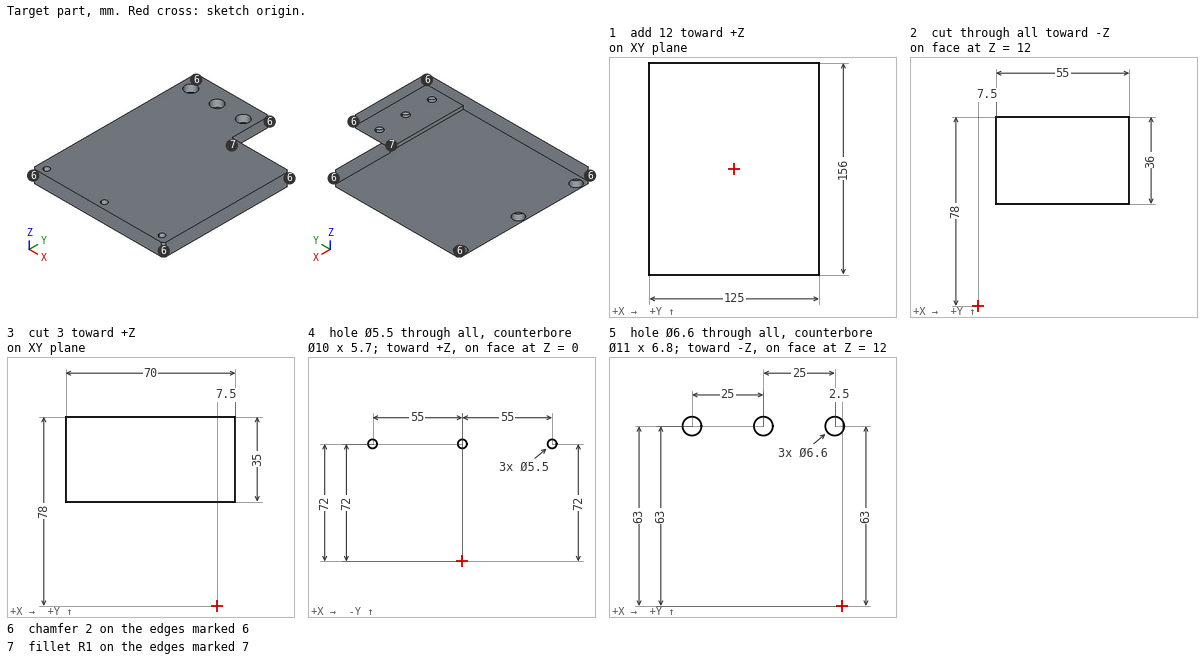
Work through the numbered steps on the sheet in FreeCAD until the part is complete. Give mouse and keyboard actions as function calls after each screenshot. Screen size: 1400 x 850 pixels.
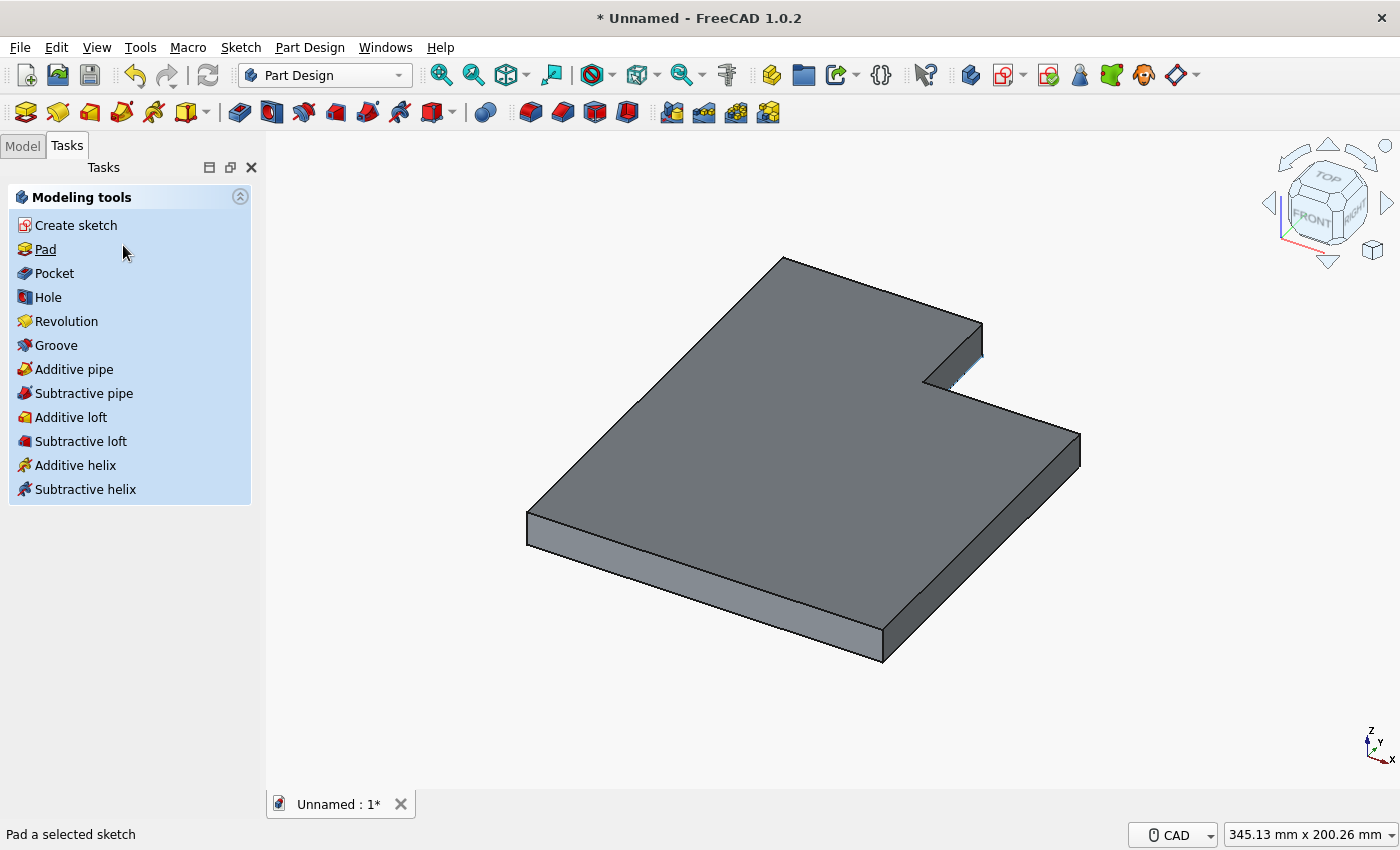
click(240, 112)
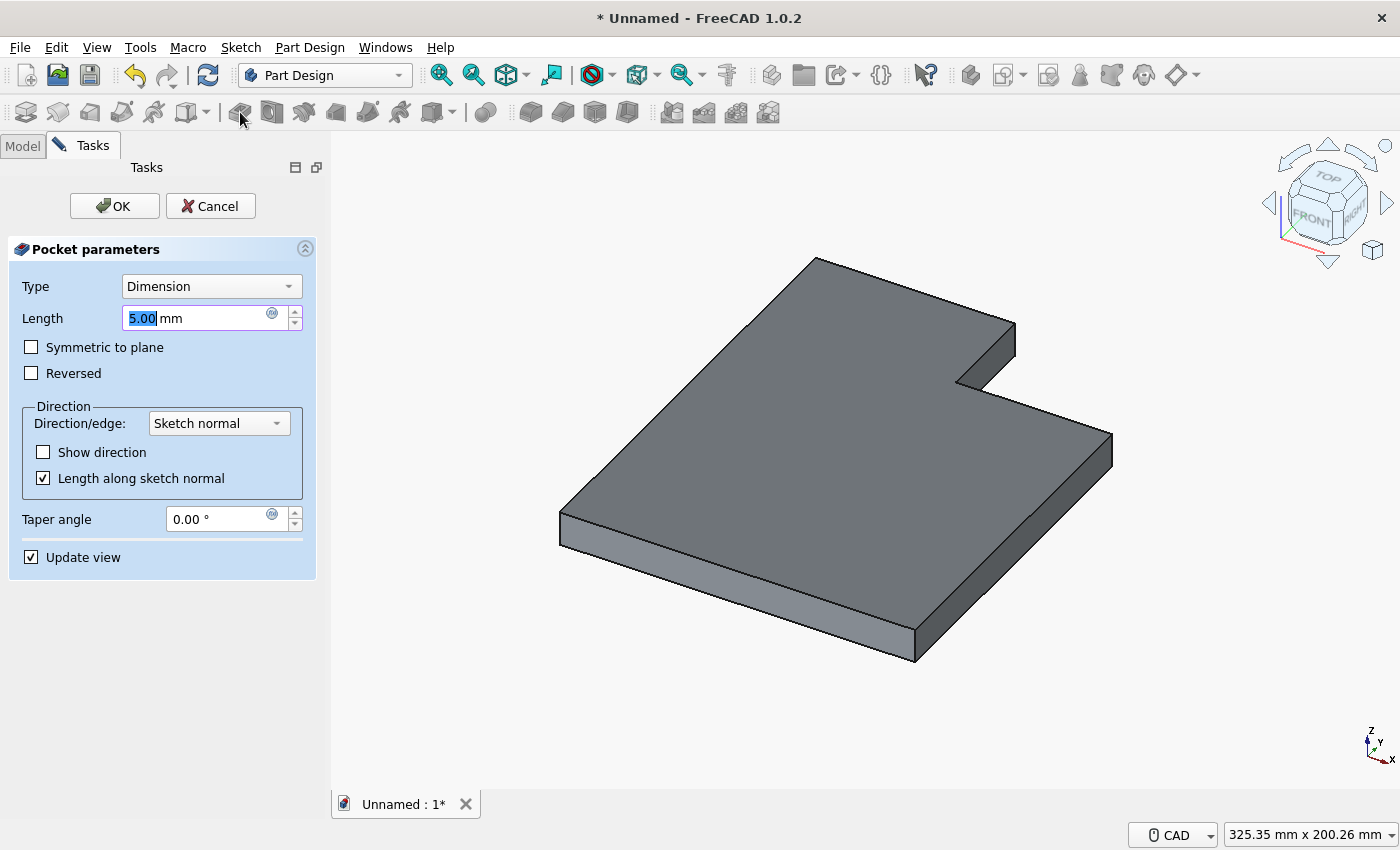
text(3)
key(Tab)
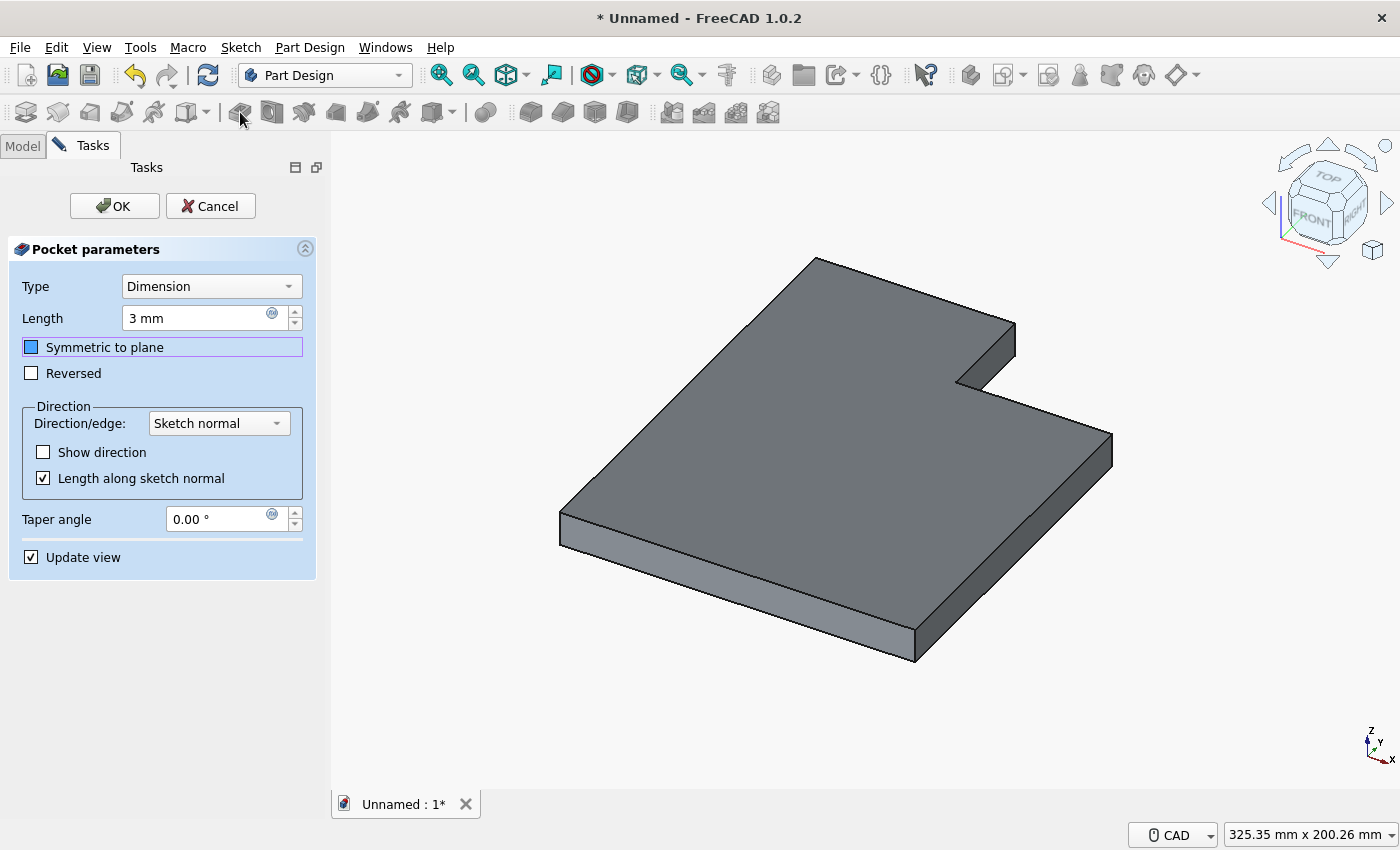
click(30, 373)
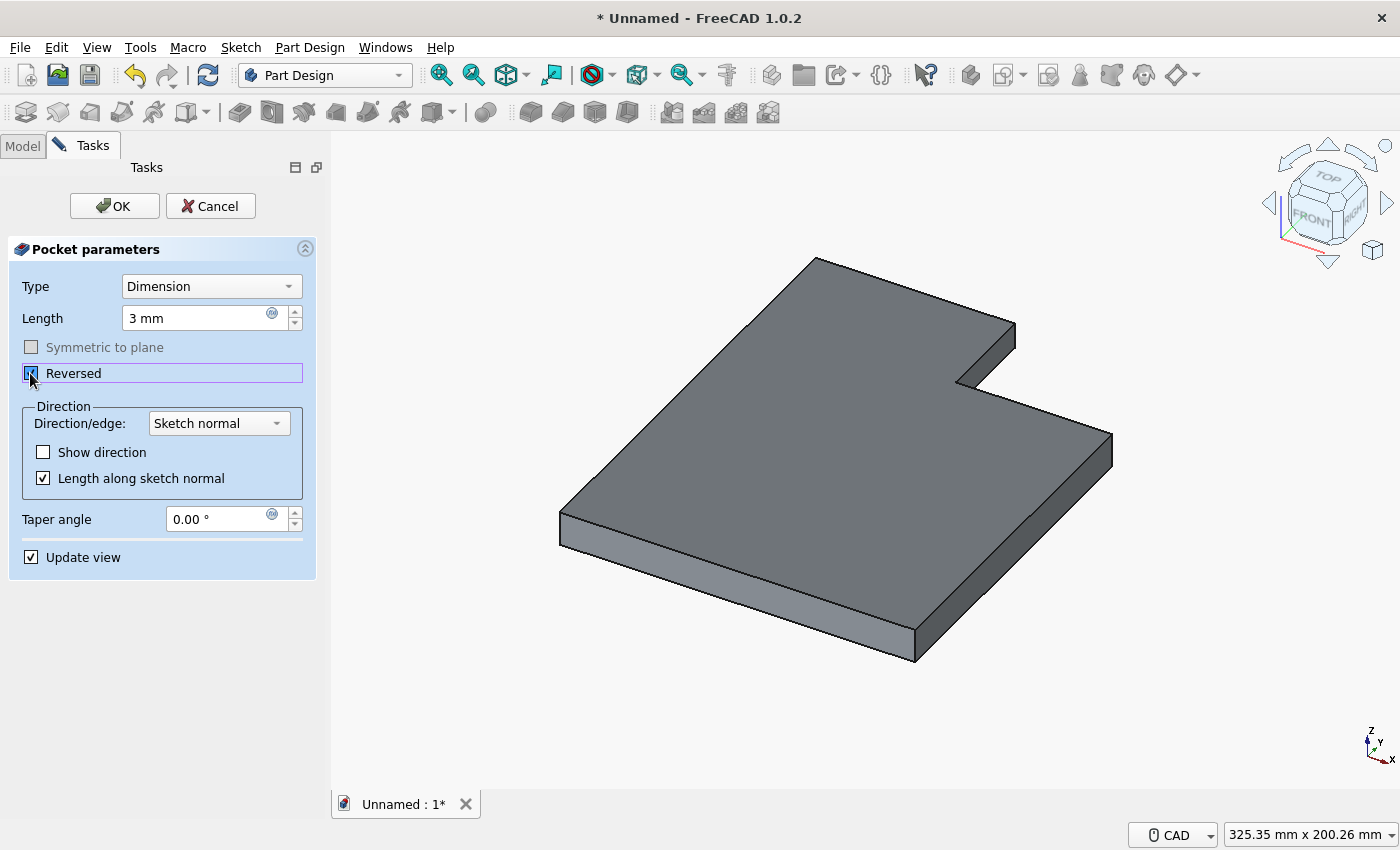
click(115, 206)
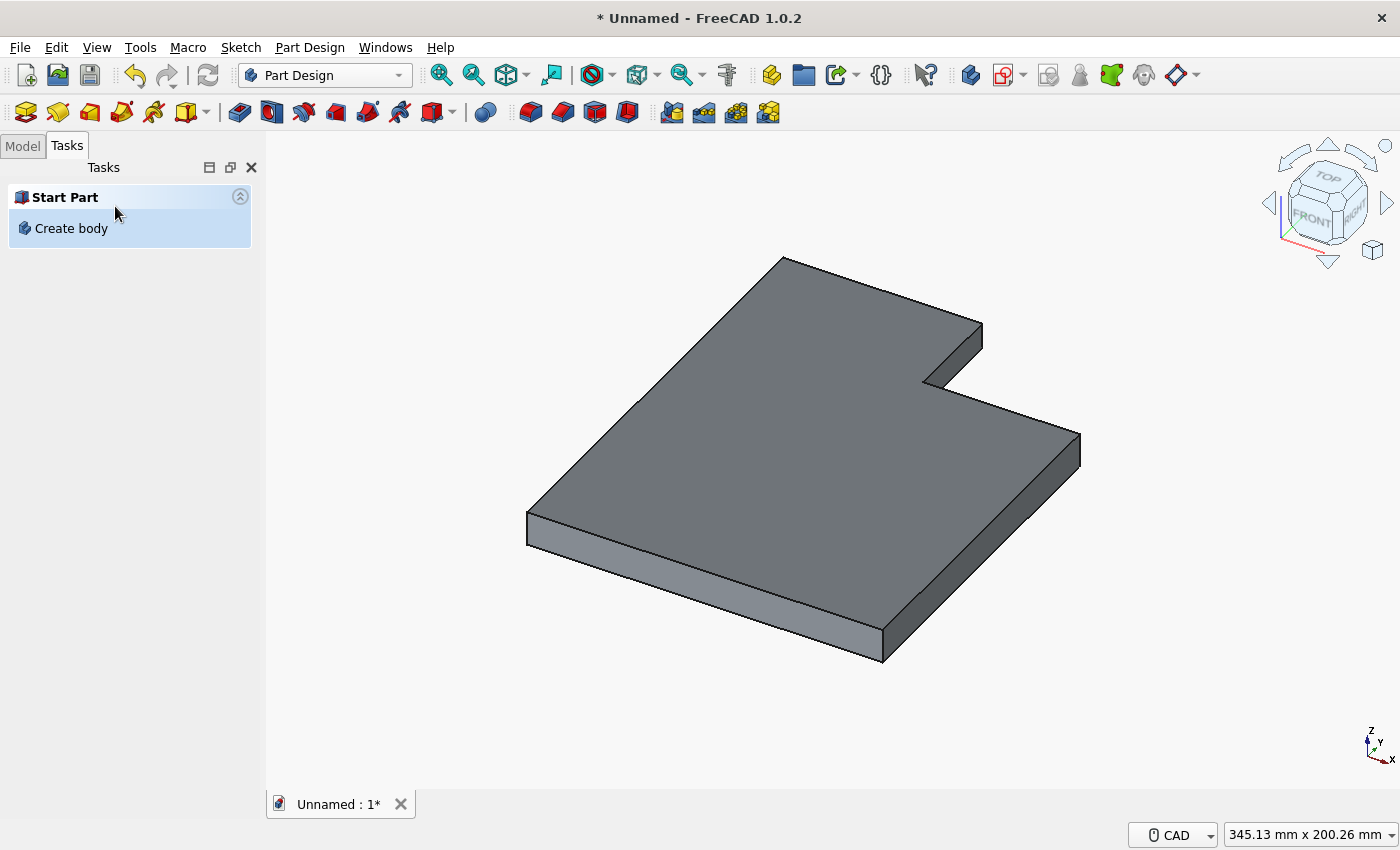
key(5)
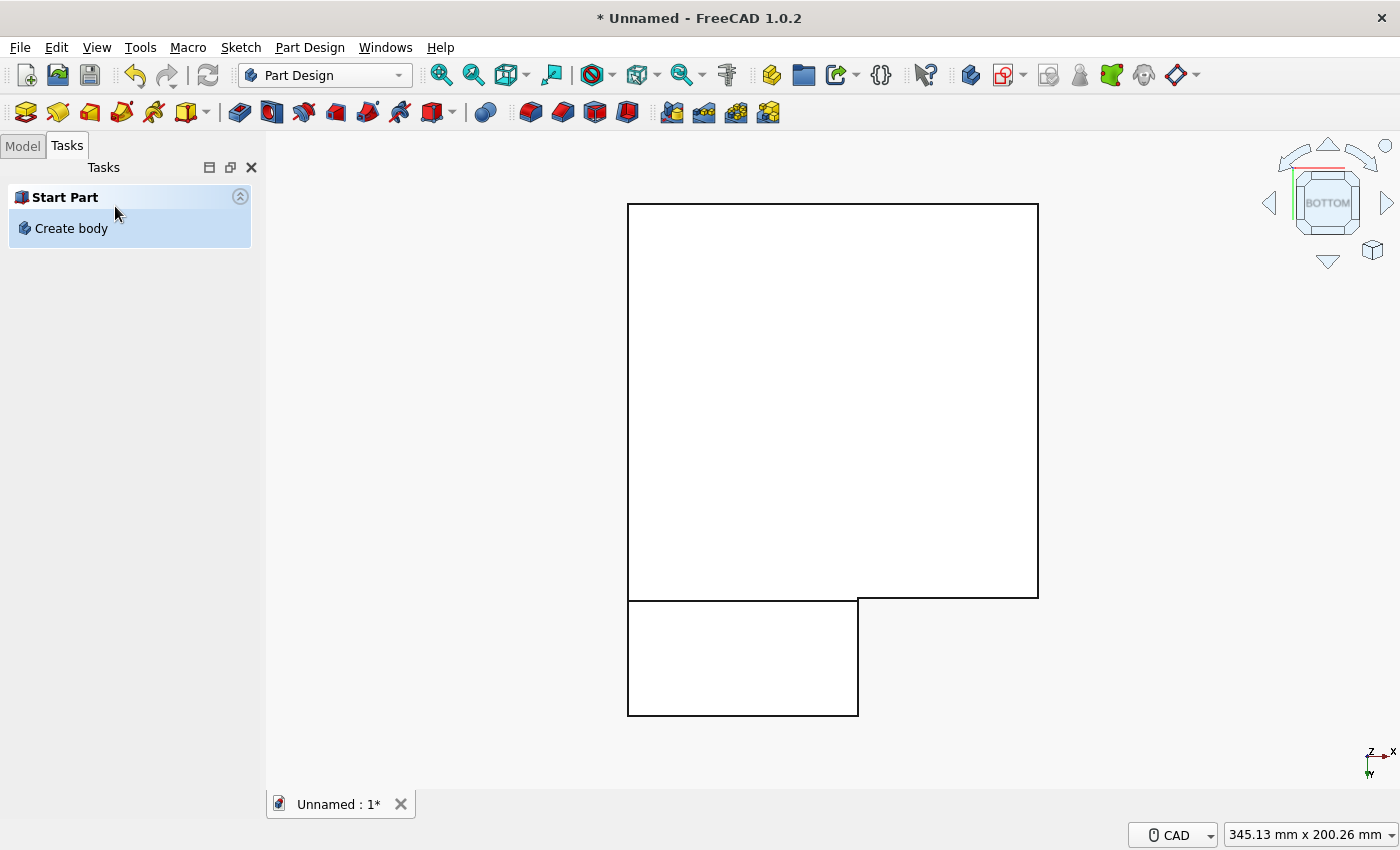
click(833, 402)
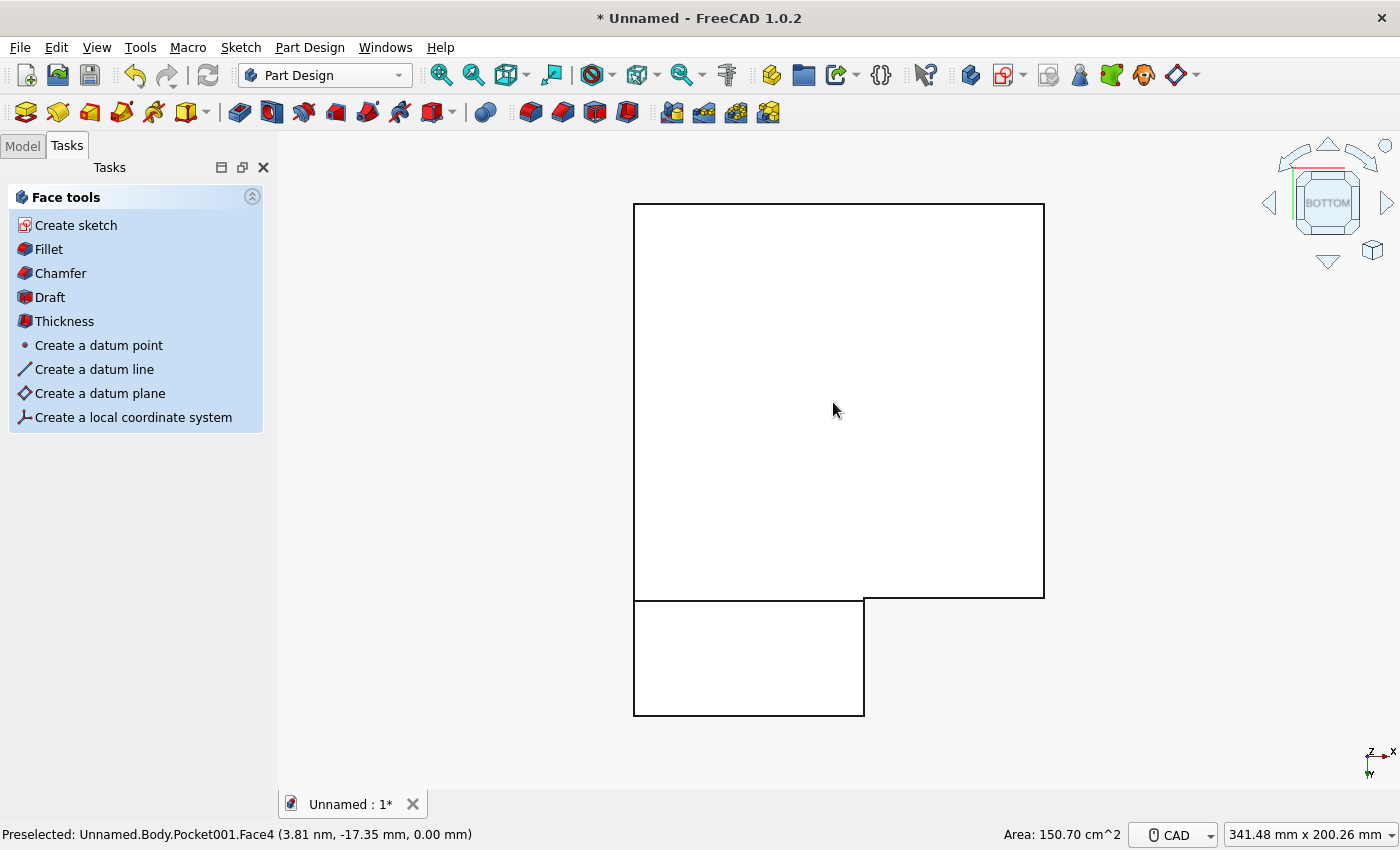
click(1004, 76)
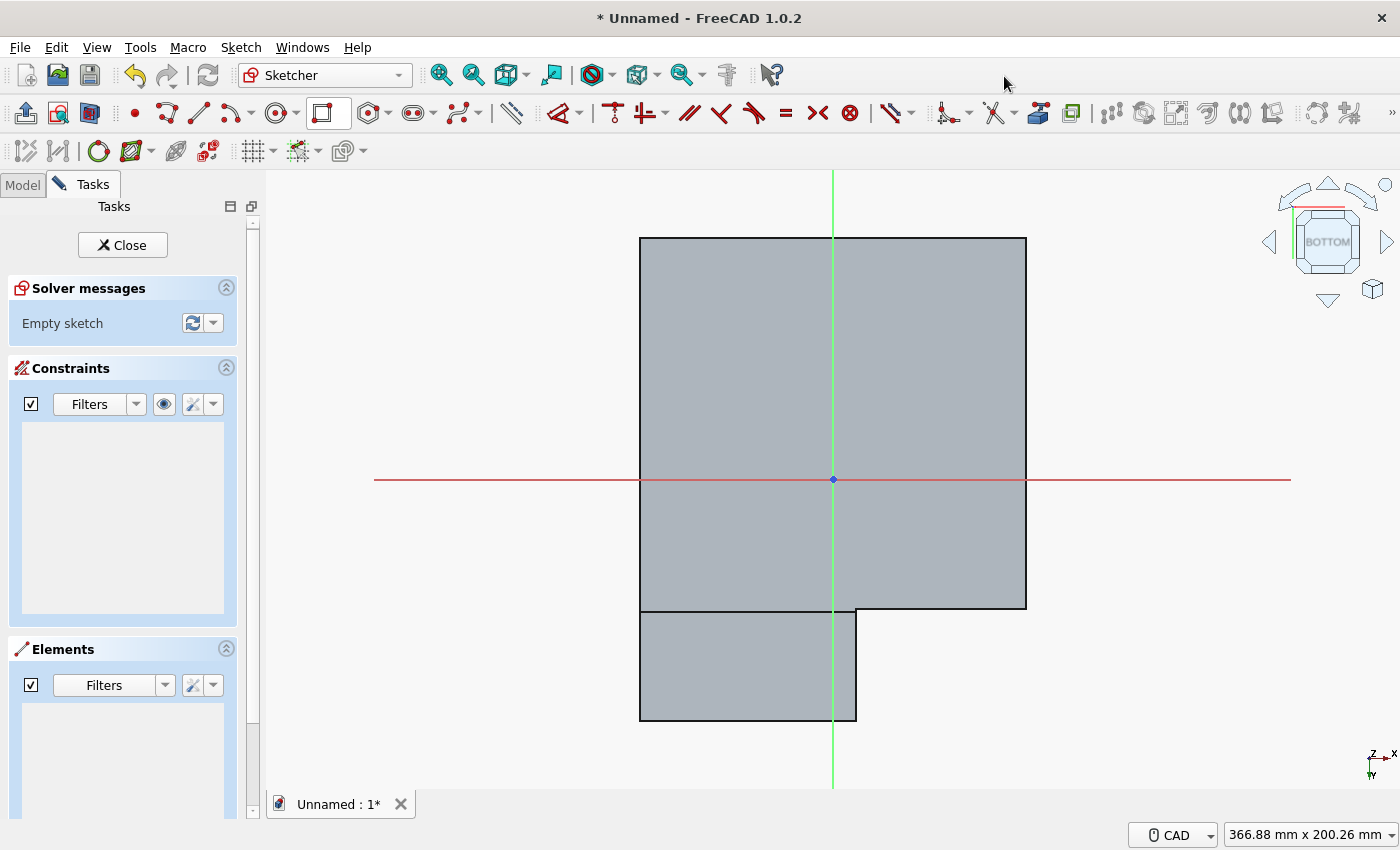
scroll(916, 223, up, 3)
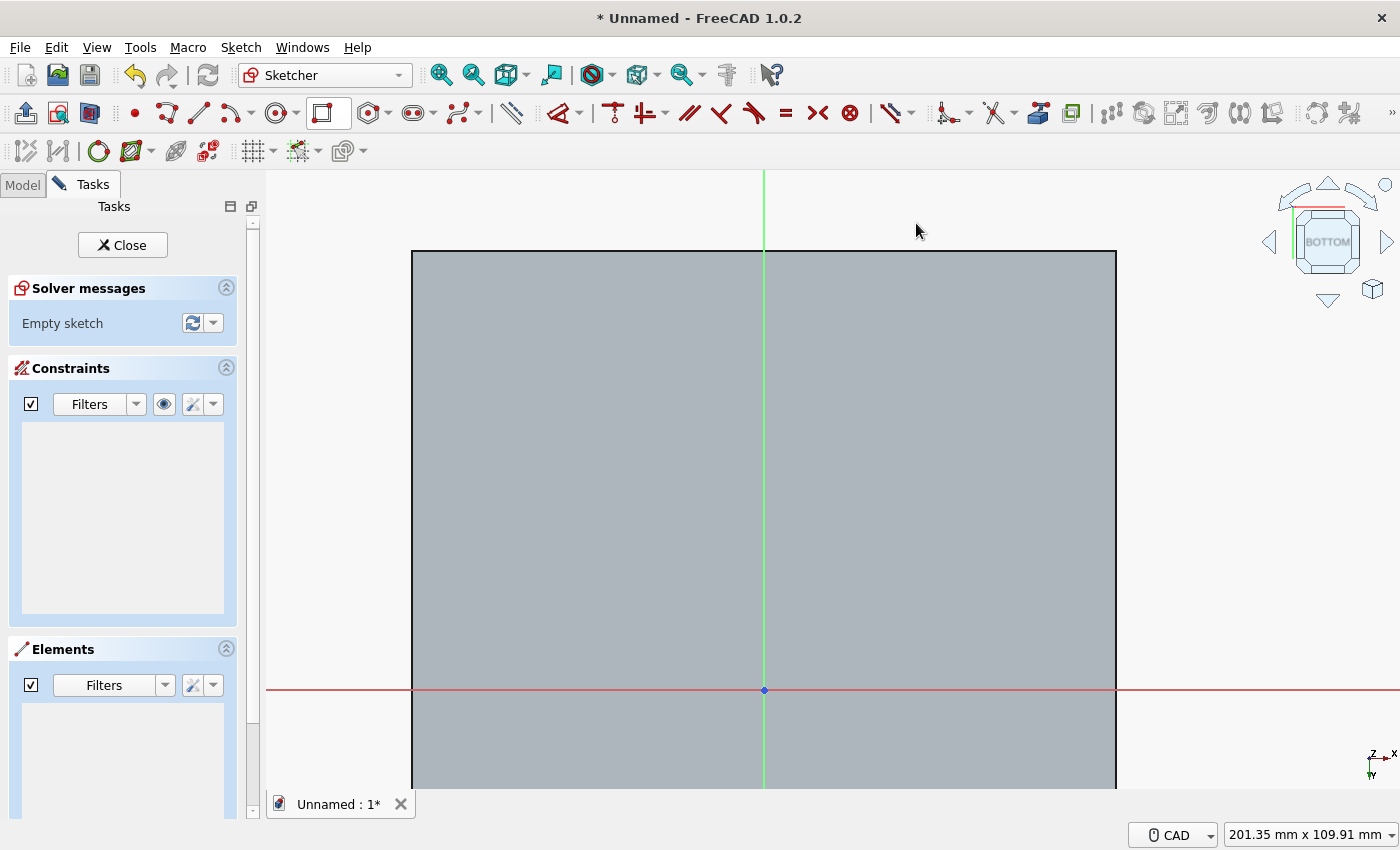
click(276, 114)